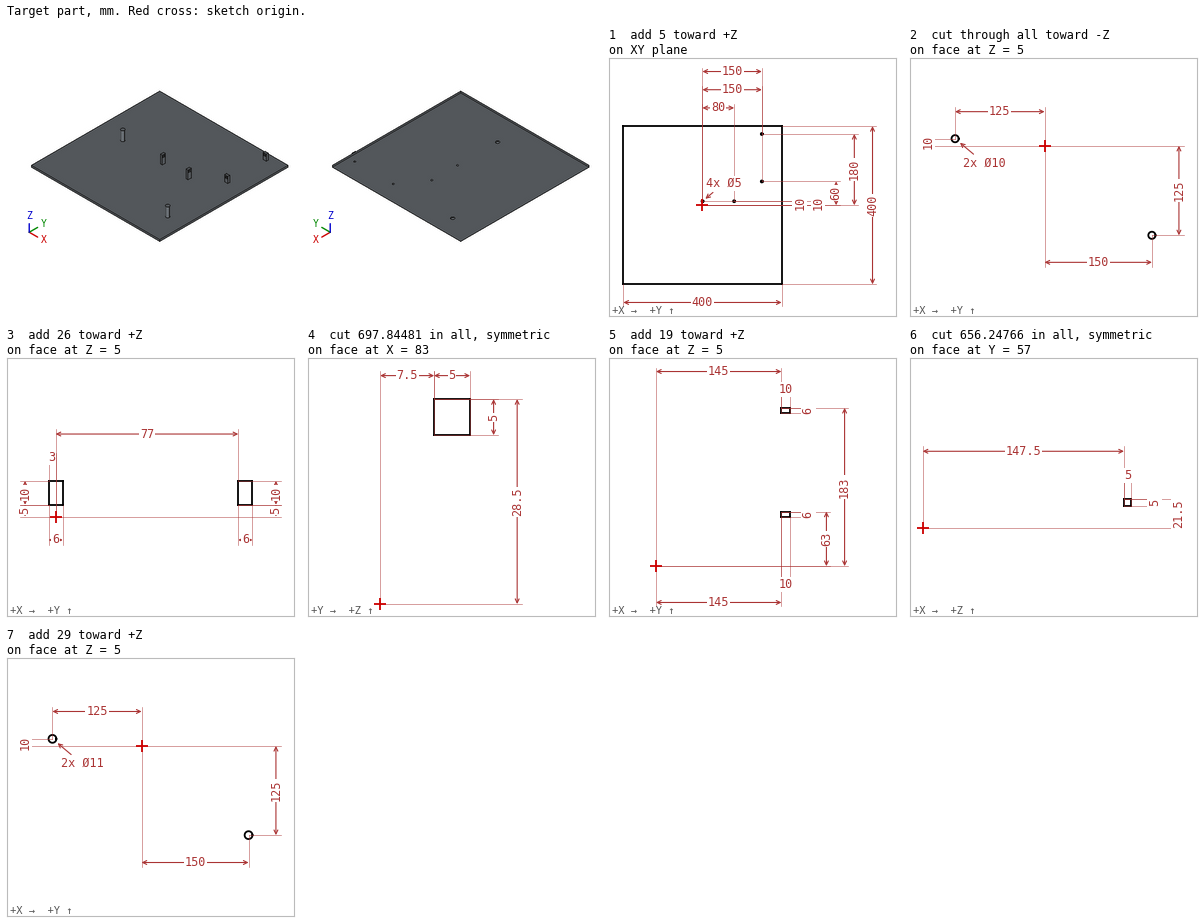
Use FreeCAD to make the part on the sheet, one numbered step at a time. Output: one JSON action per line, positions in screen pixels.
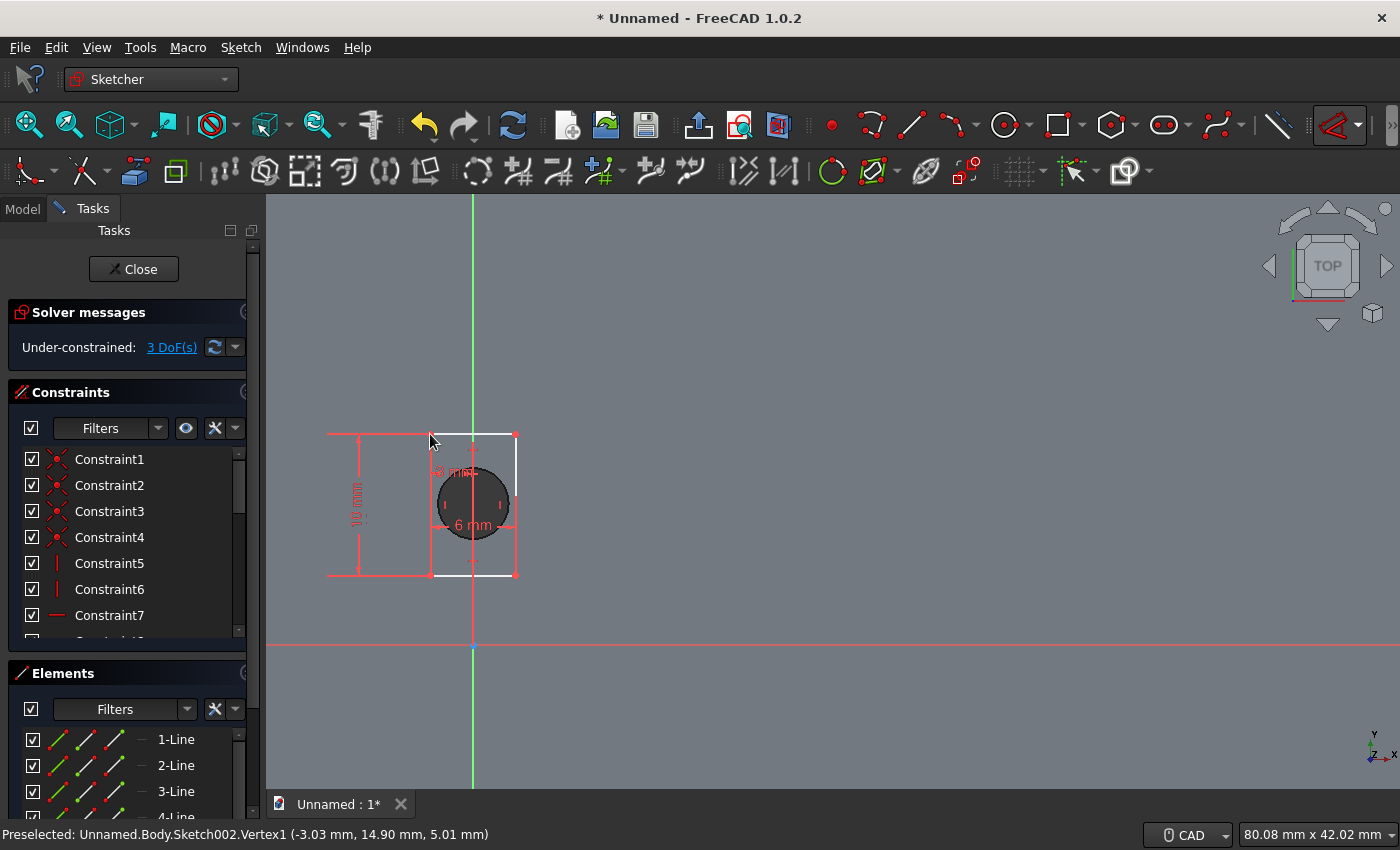
{"action": "left_click", "coordinate": [431, 576]}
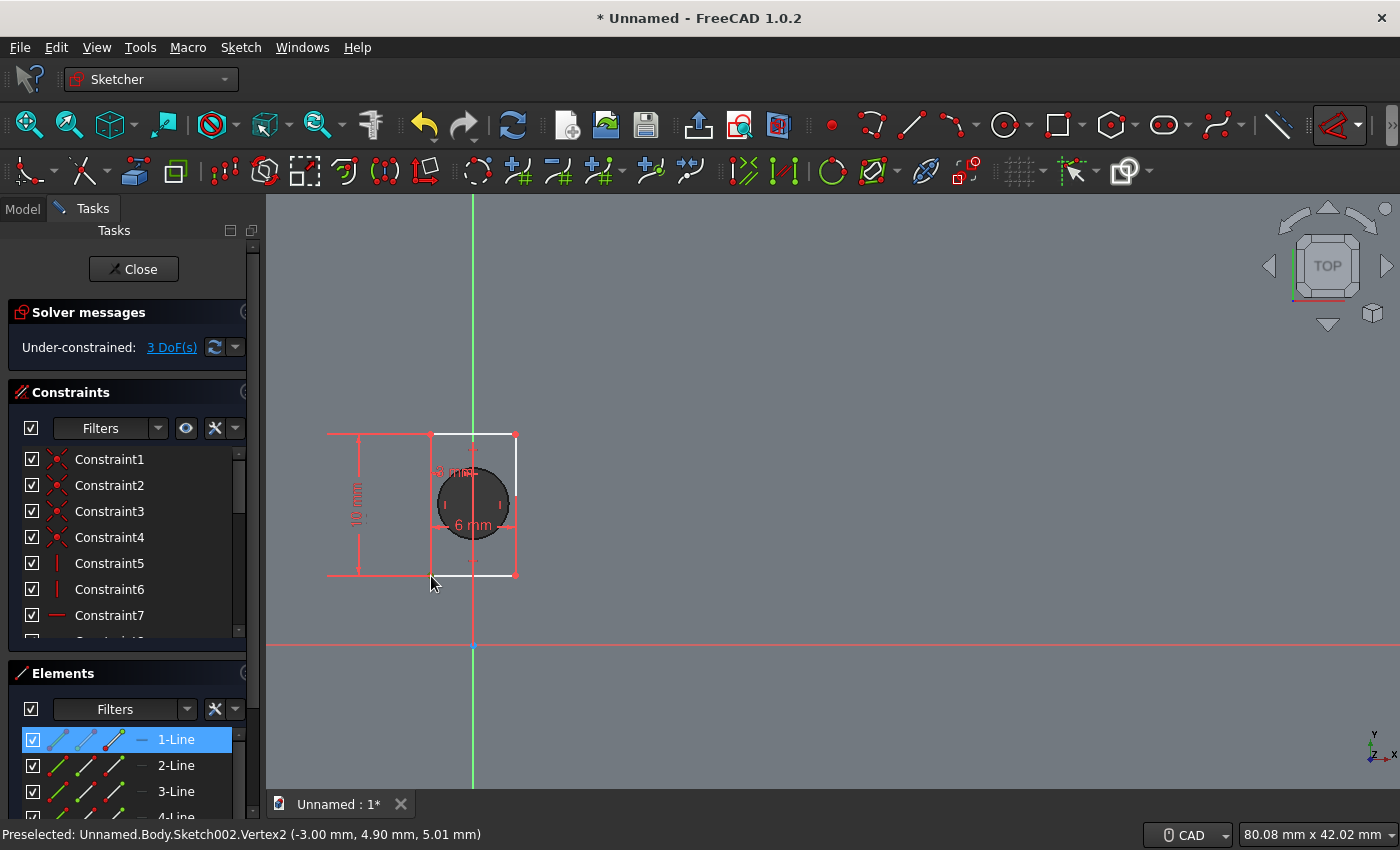
{"action": "key", "text": "i"}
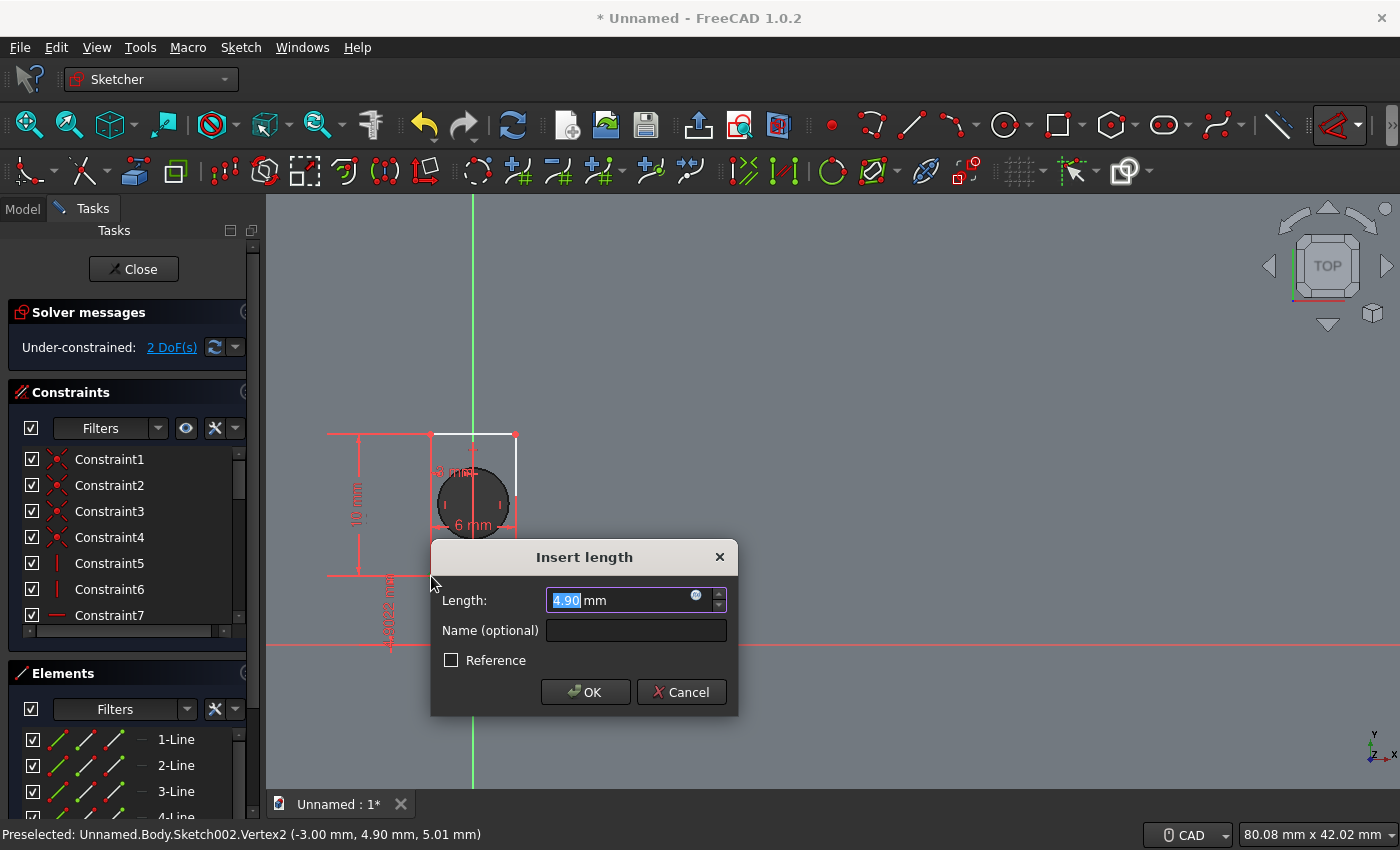
{"action": "type", "text": "5"}
{"action": "key", "text": "Return"}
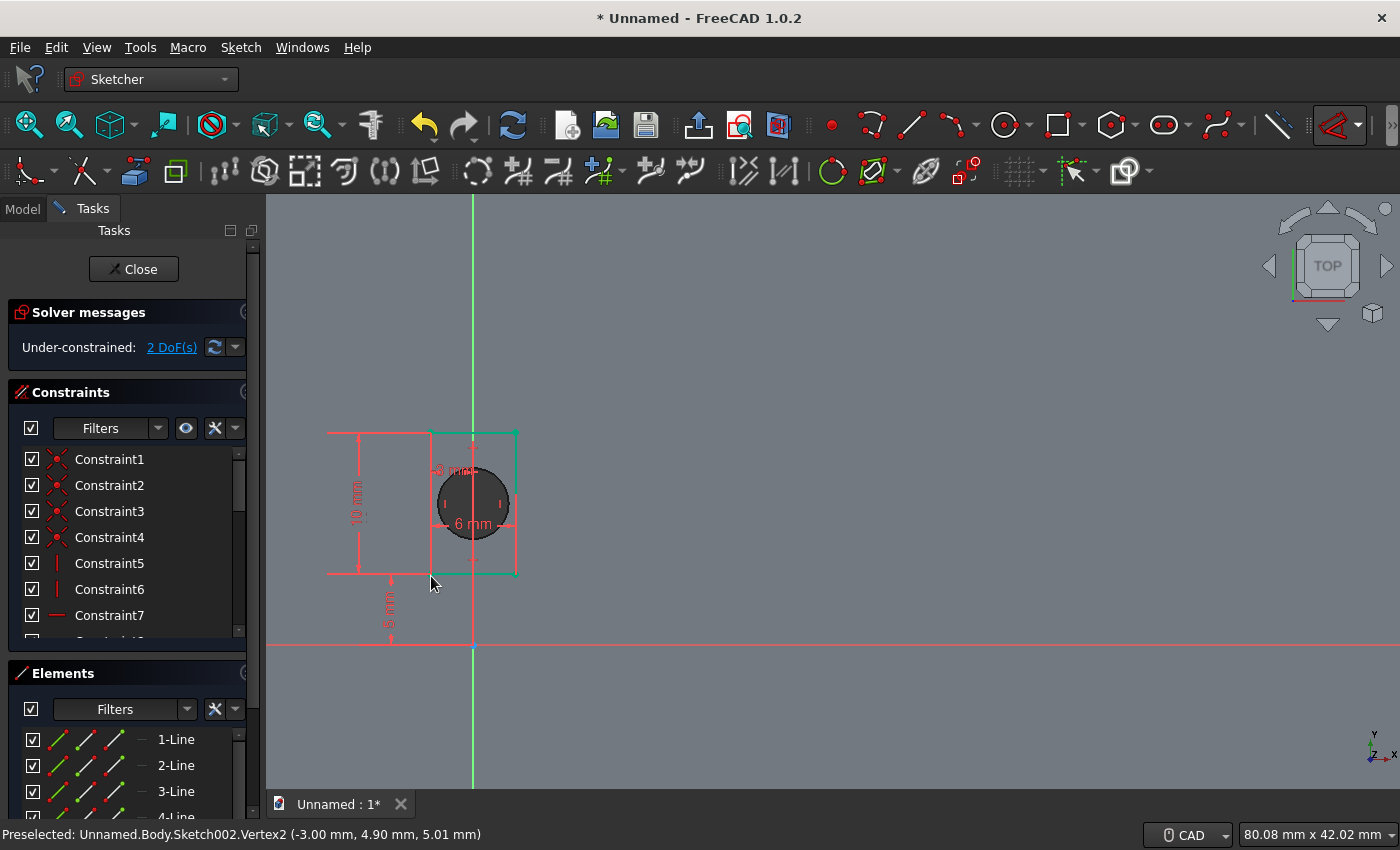
{"action": "scroll", "coordinate": [430, 434], "scroll_direction": "down", "scroll_amount": 3}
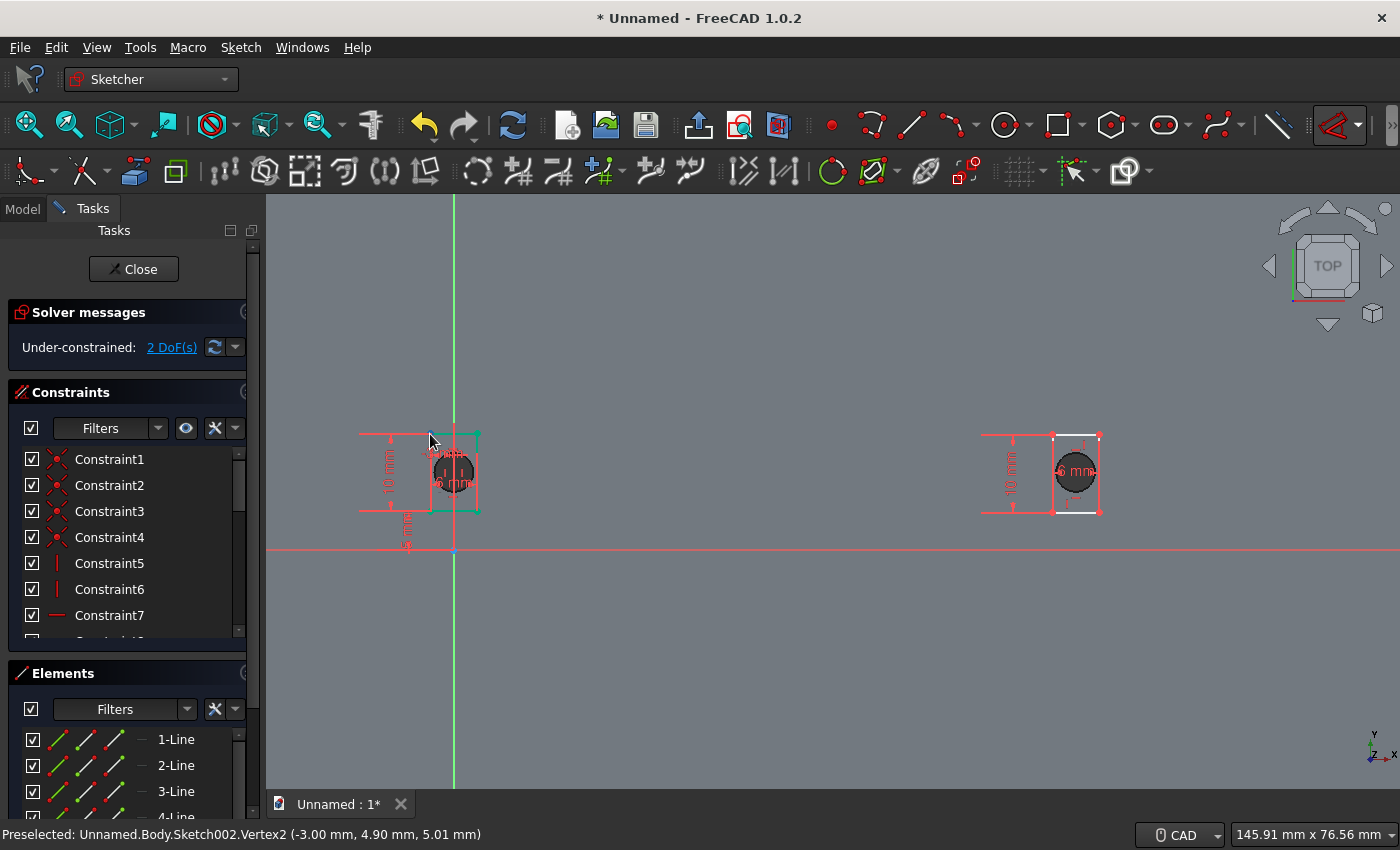
{"action": "left_click", "coordinate": [1053, 513]}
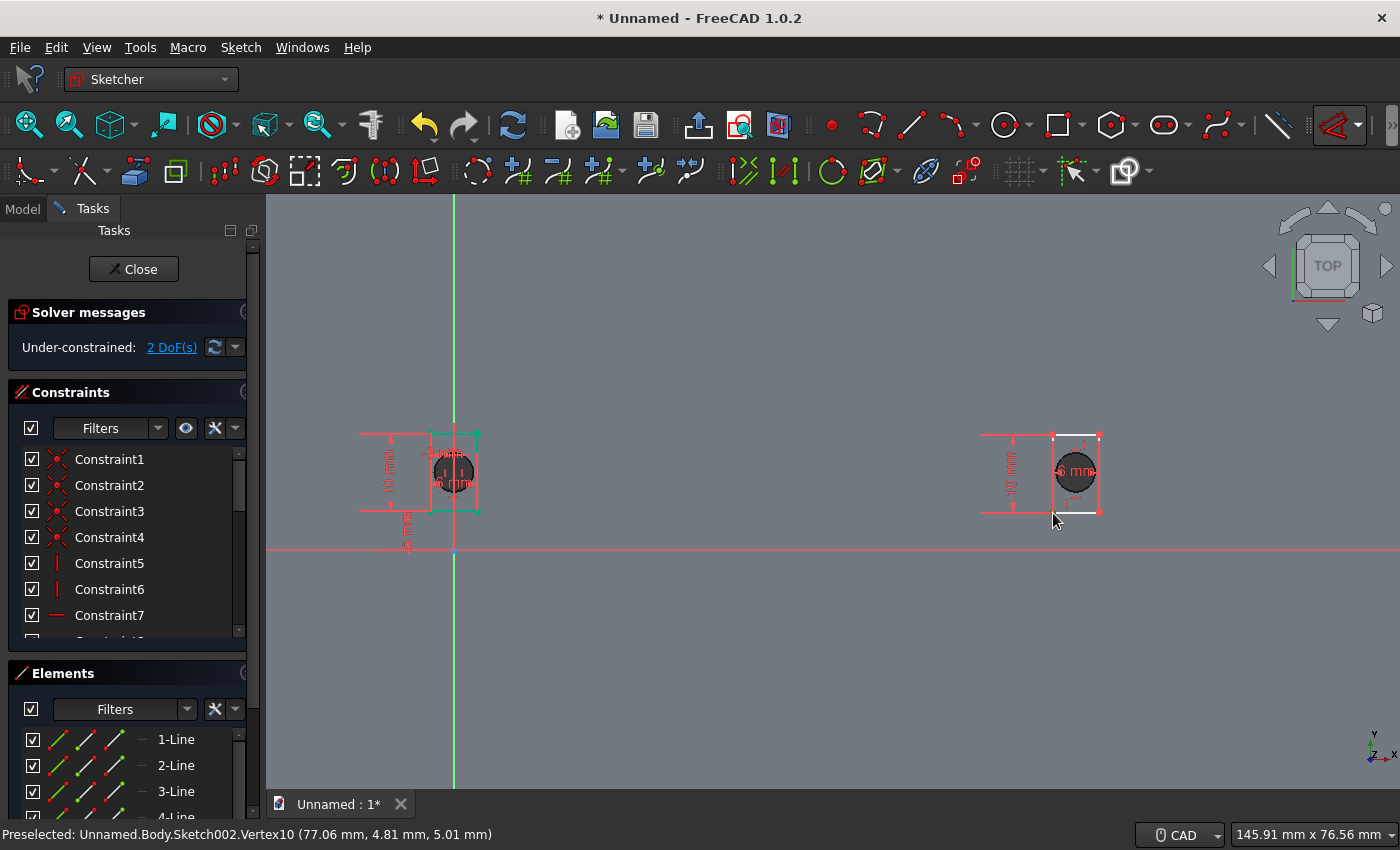
{"action": "left_click", "coordinate": [1360, 126]}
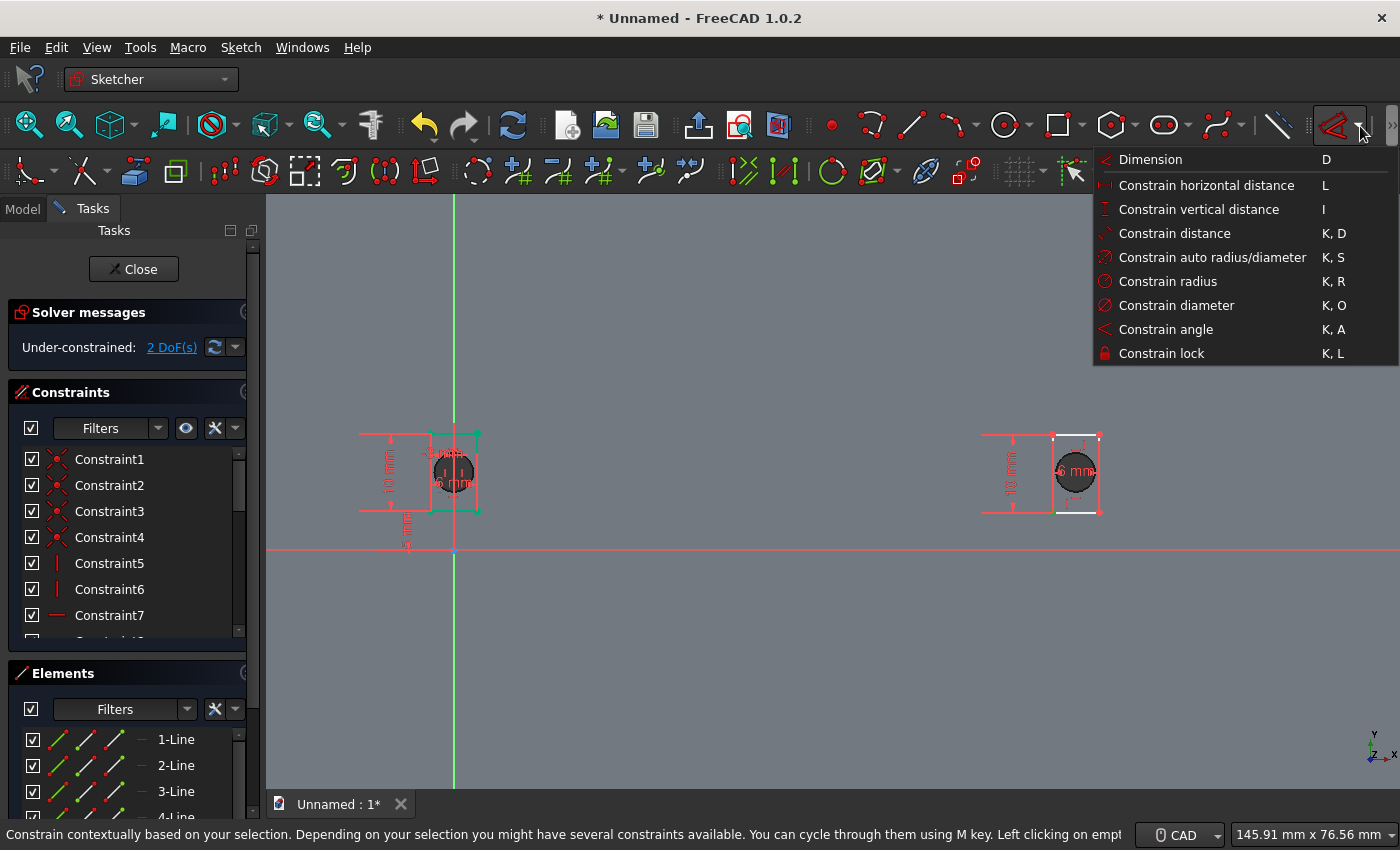
{"action": "left_click", "coordinate": [1246, 209]}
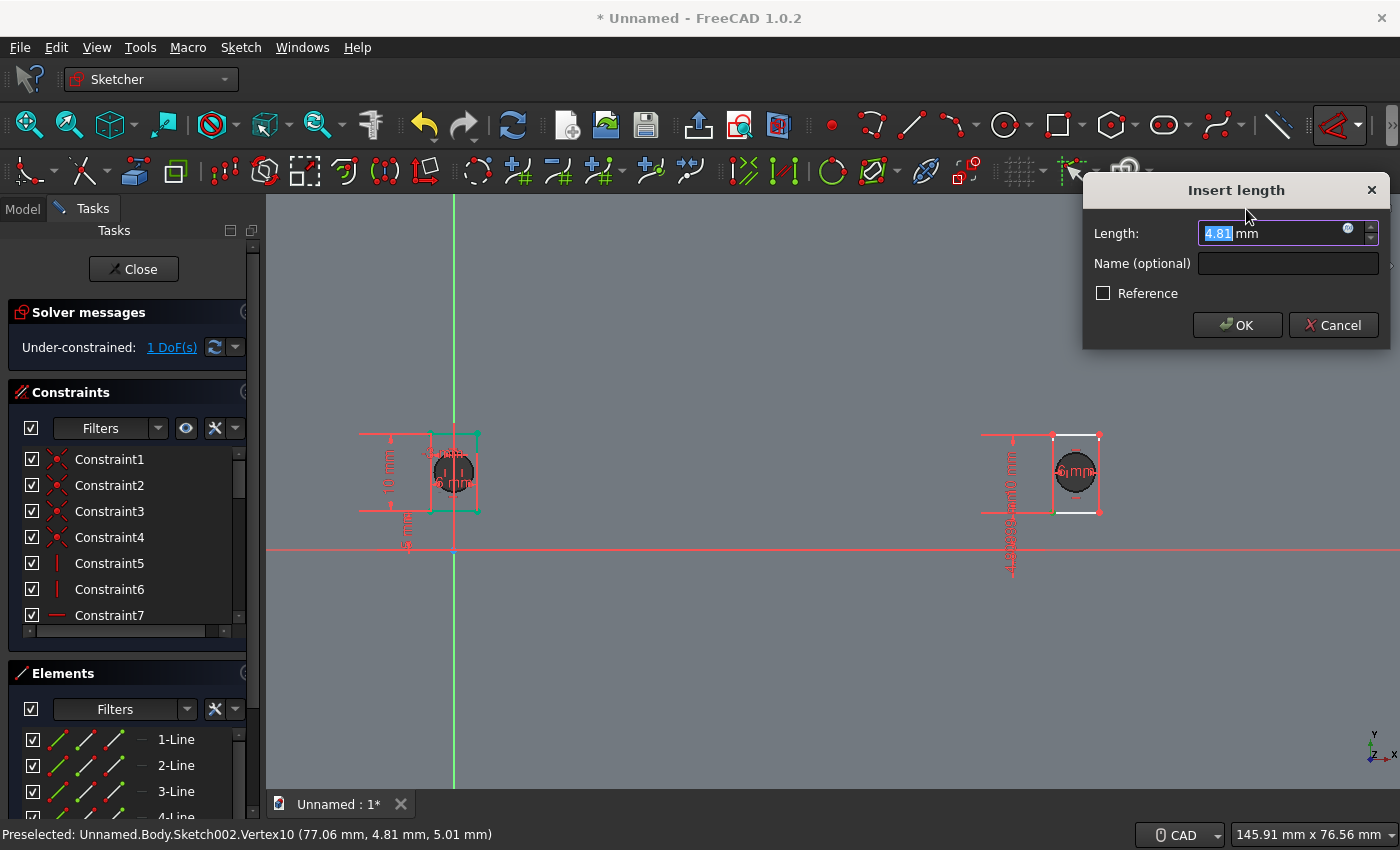
{"action": "type", "text": "5"}
{"action": "key", "text": "Return"}